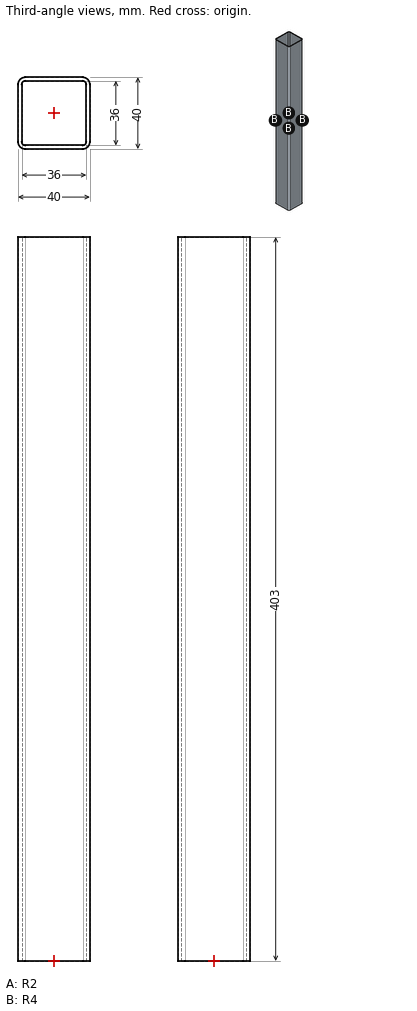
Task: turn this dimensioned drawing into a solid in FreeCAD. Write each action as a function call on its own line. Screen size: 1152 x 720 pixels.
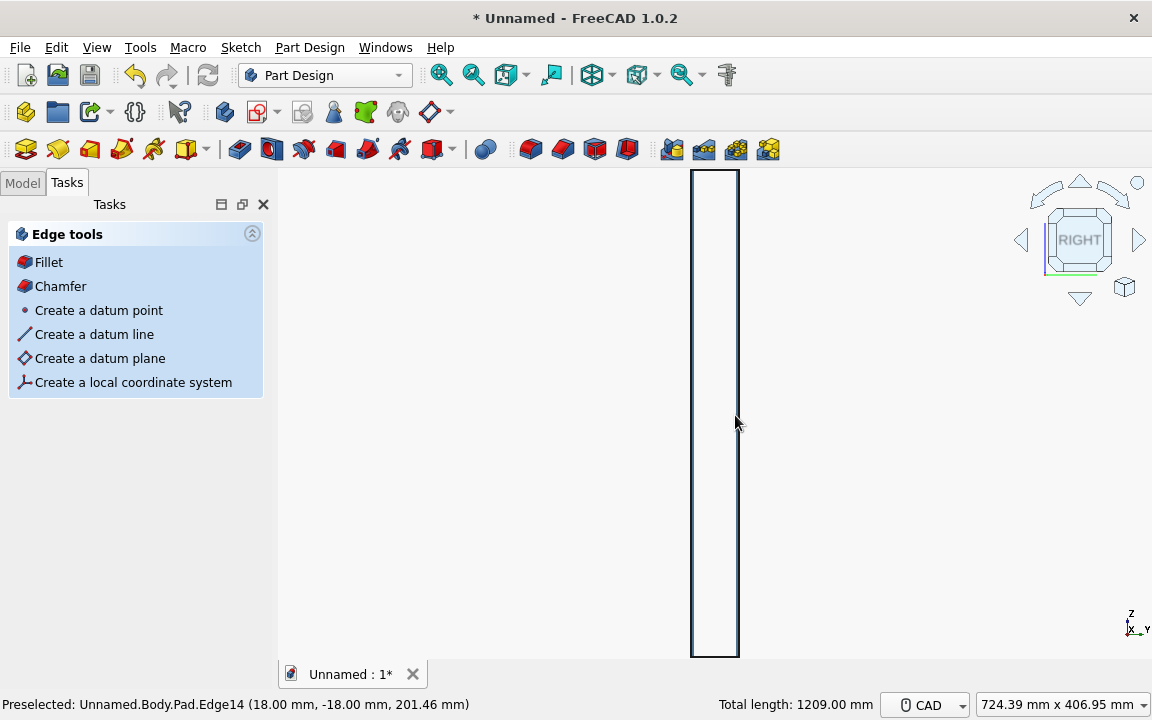
scroll(737, 412, up, 6)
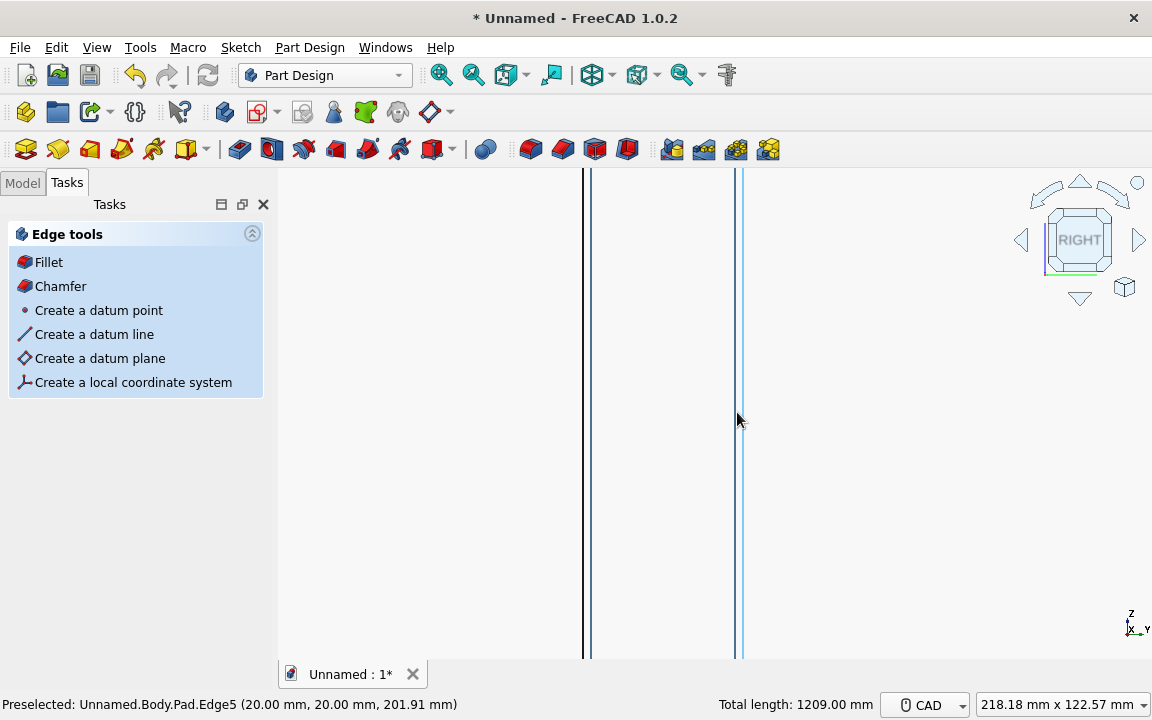
key(v)
key(f)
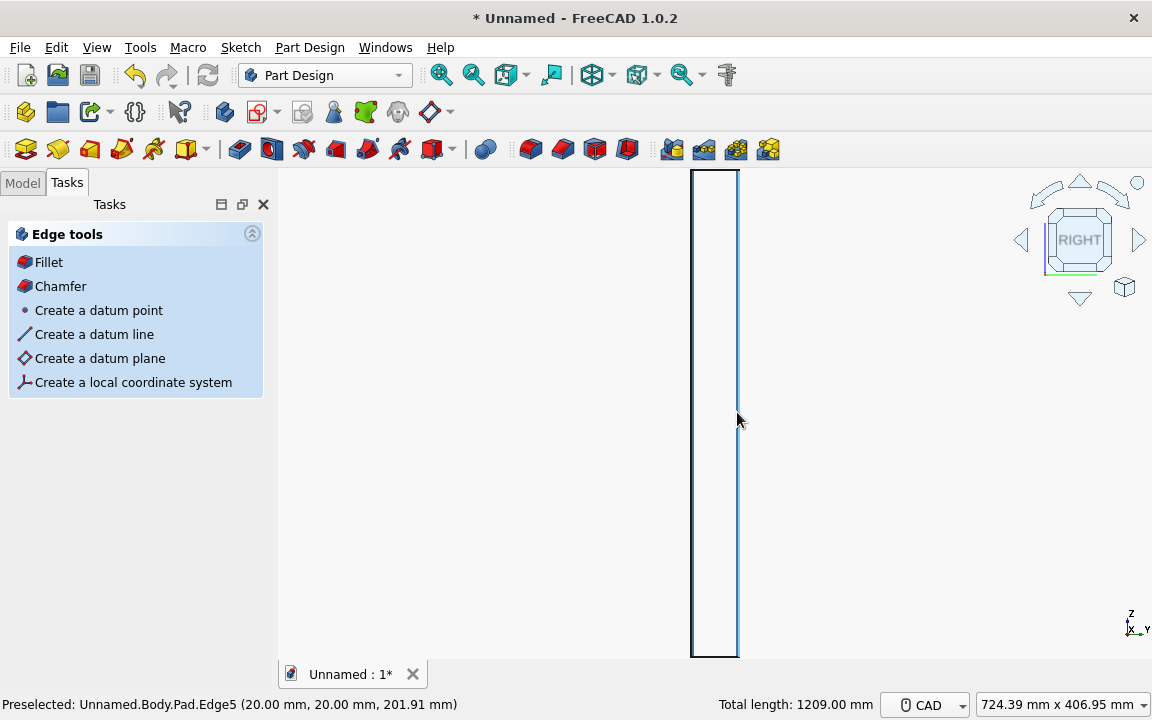
key(5)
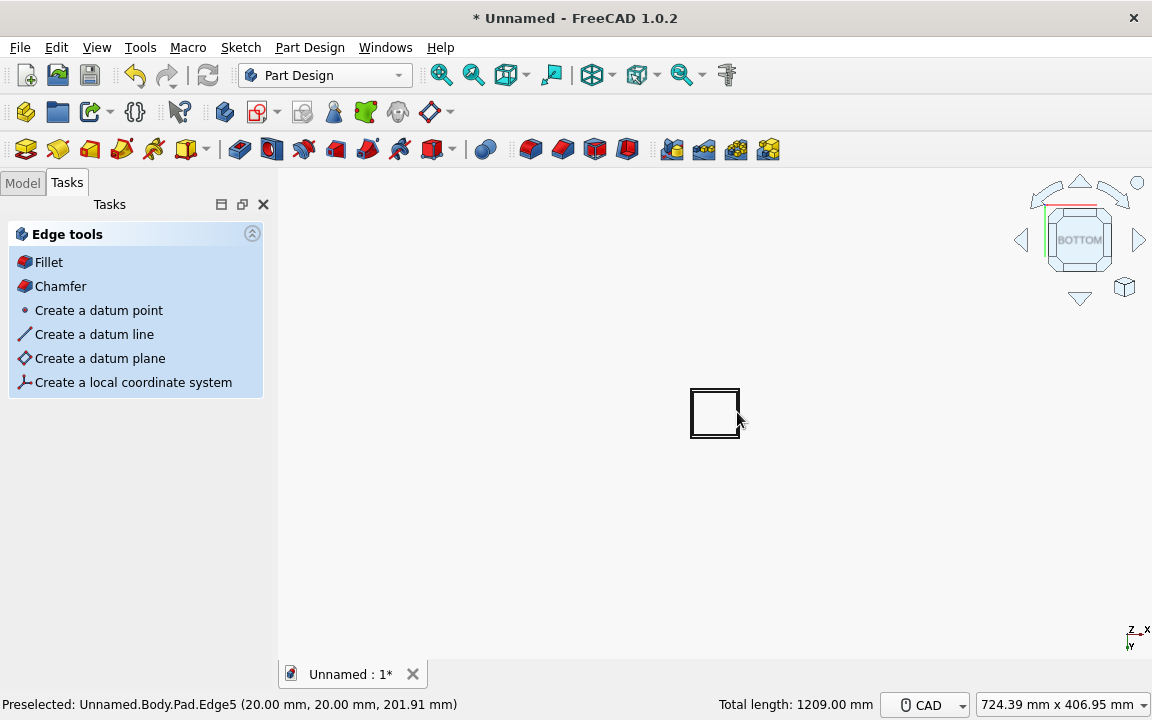
key(v)
key(f)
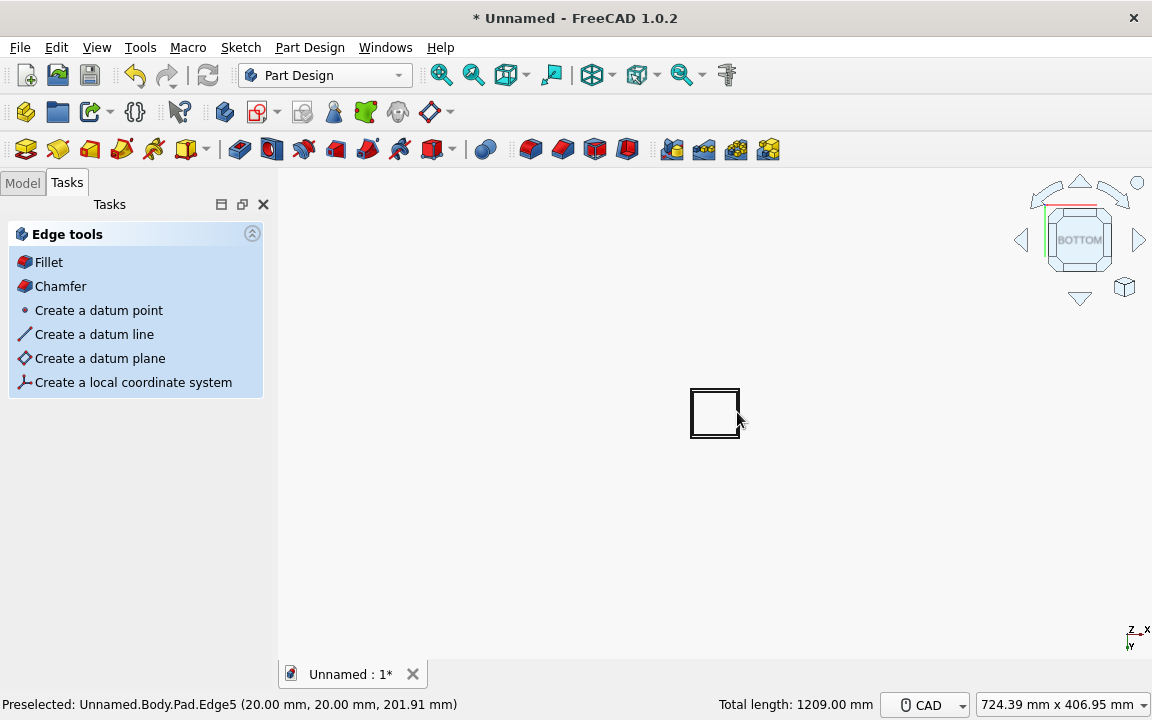
scroll(693, 434, up, 6)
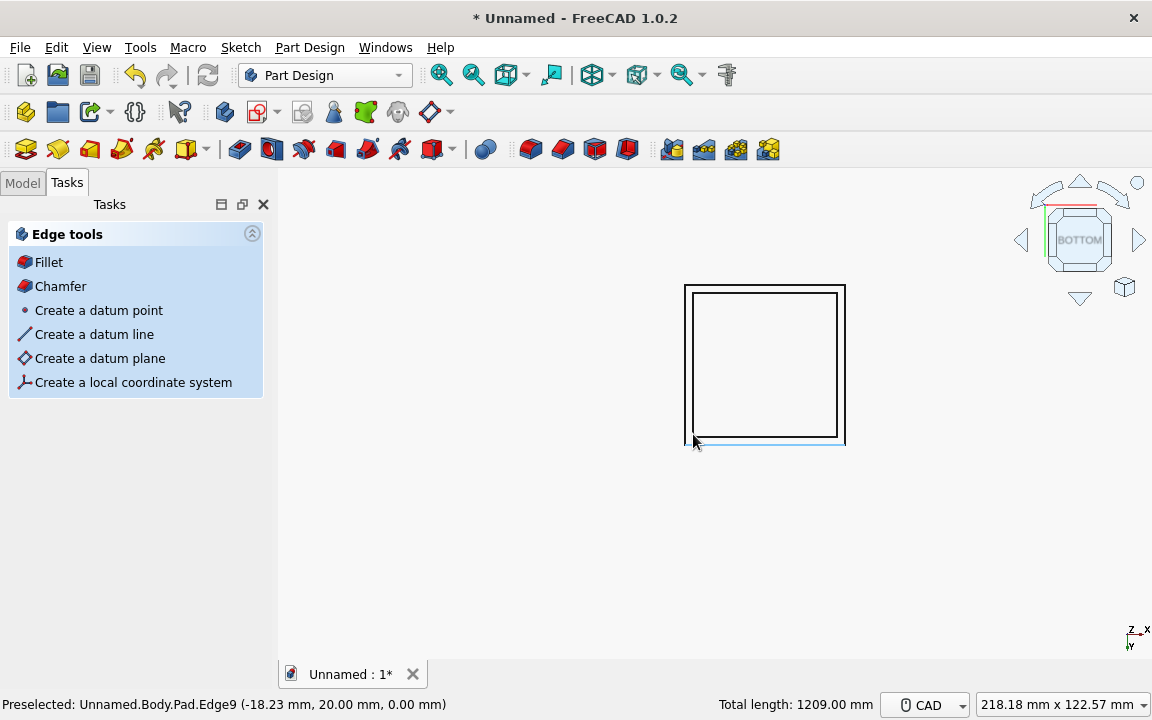
click(442, 76)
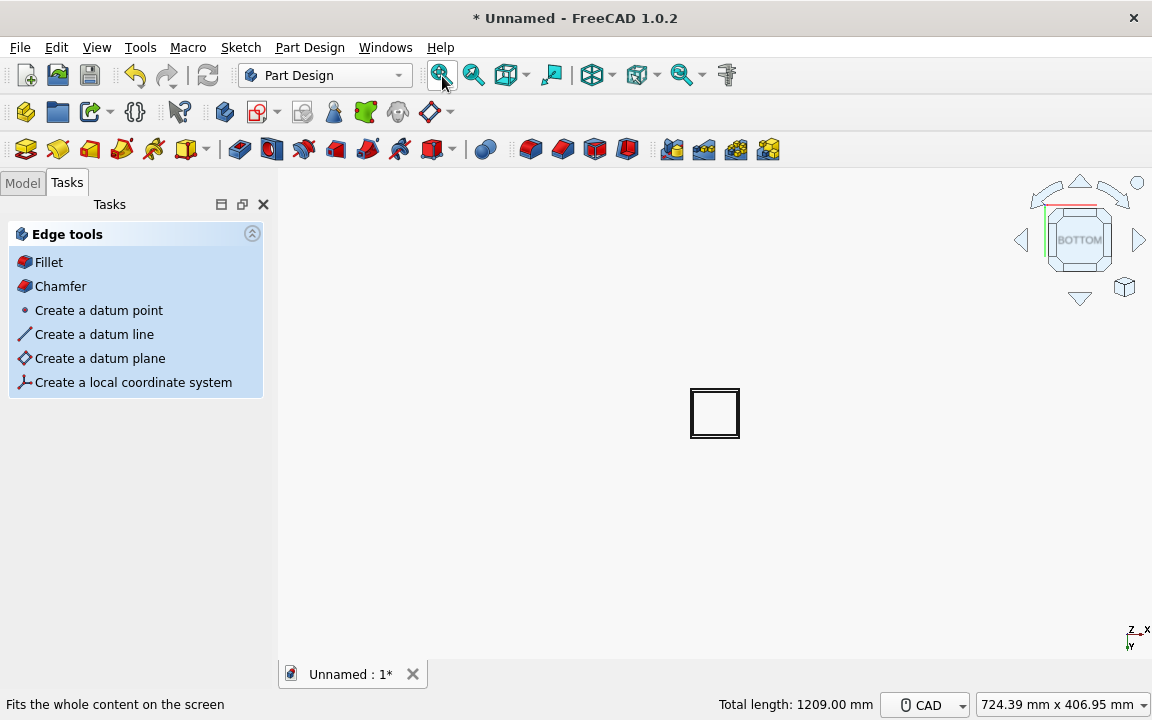
key(4)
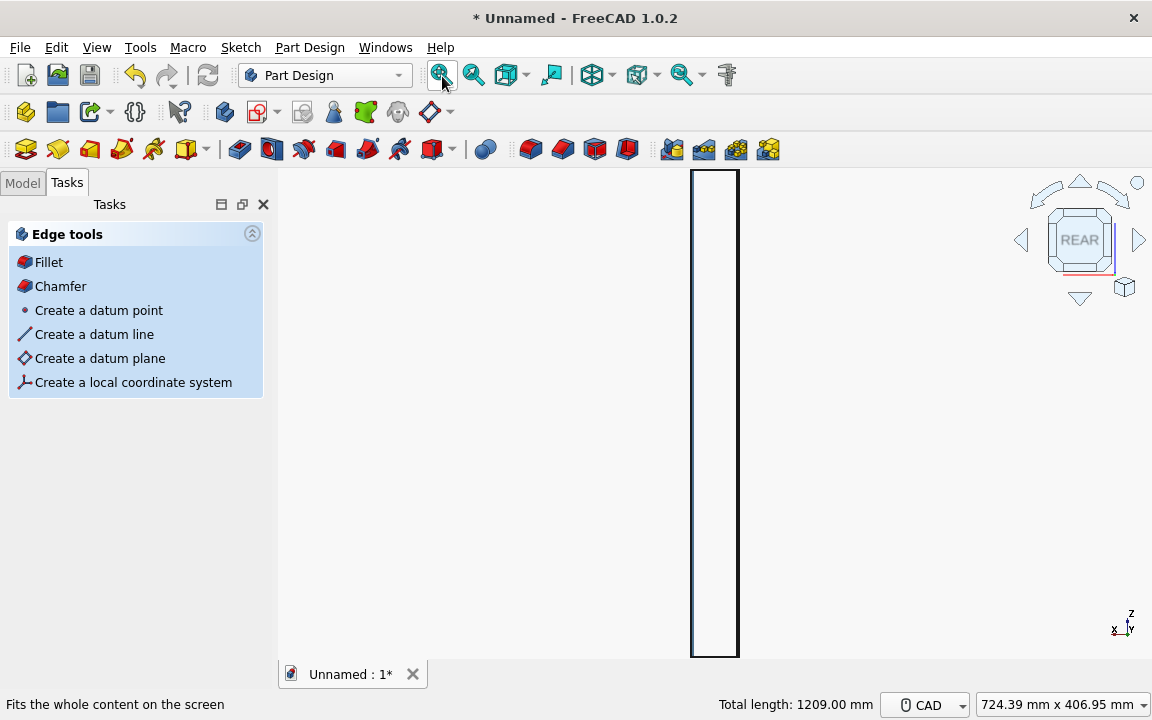
scroll(737, 412, up, 6)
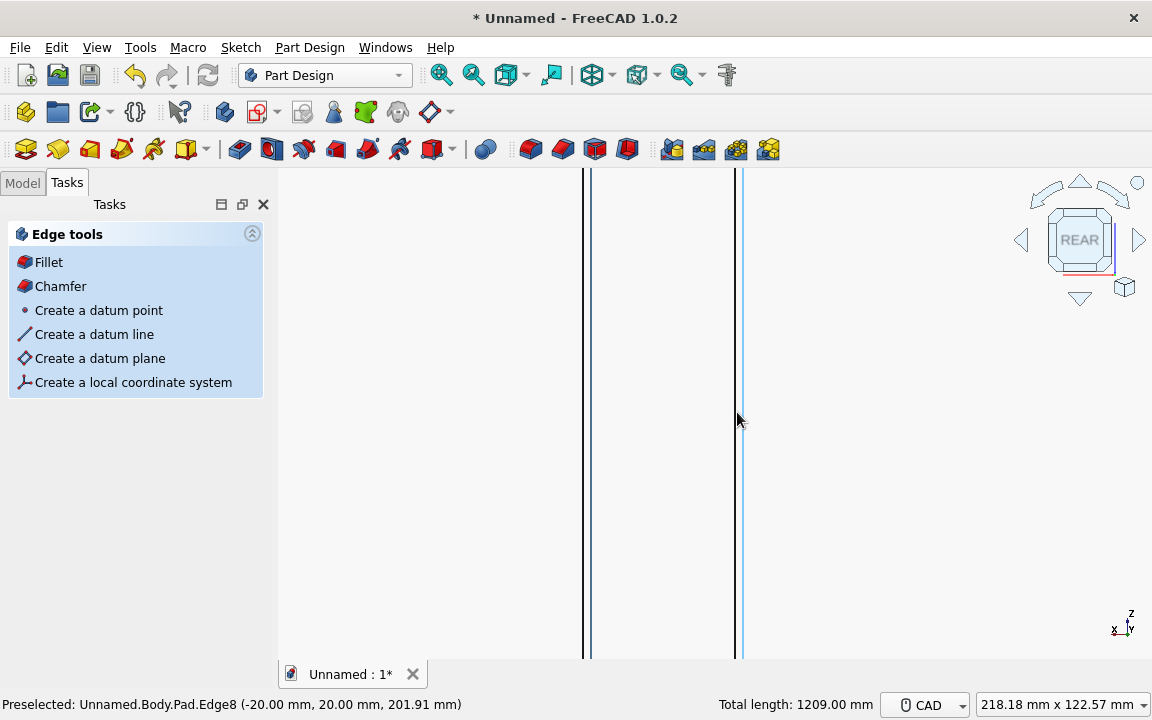
click(735, 415, ctrl)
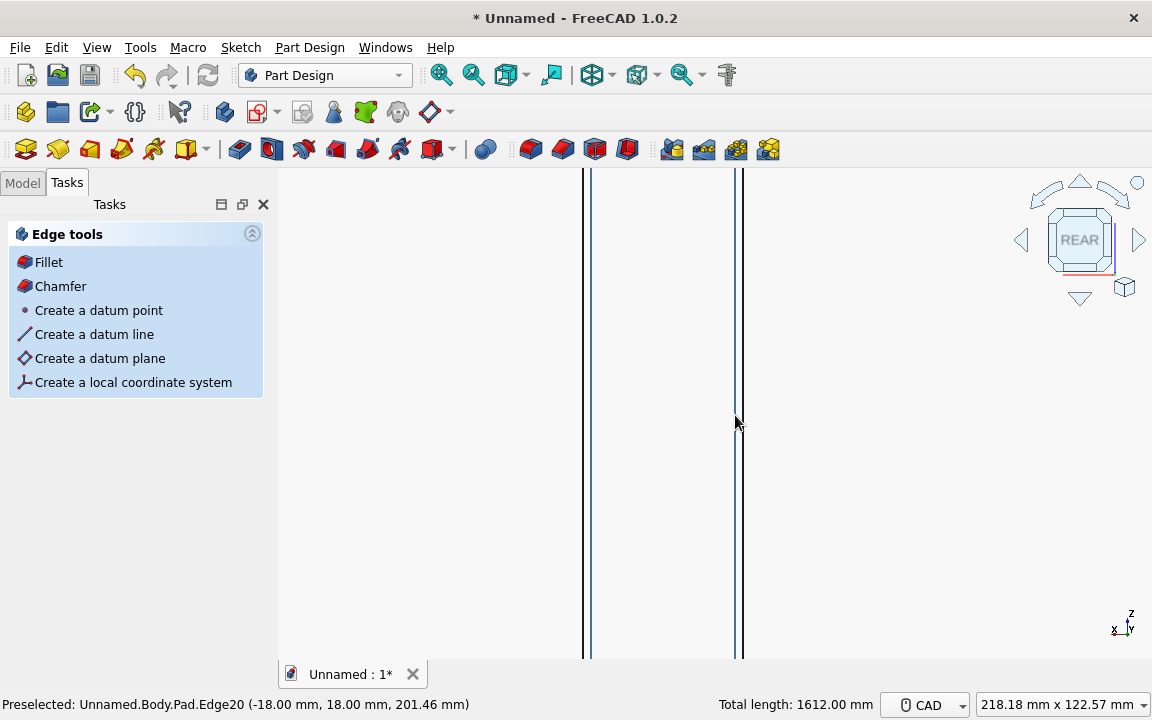
key(v)
key(1)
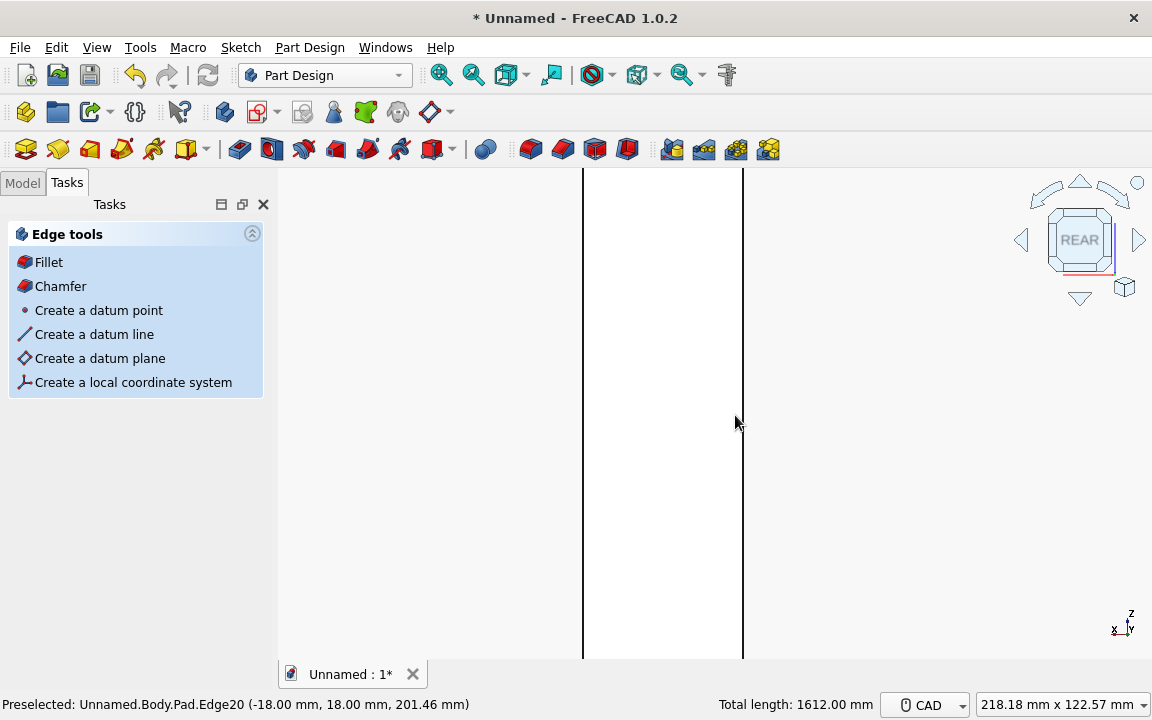
click(532, 150)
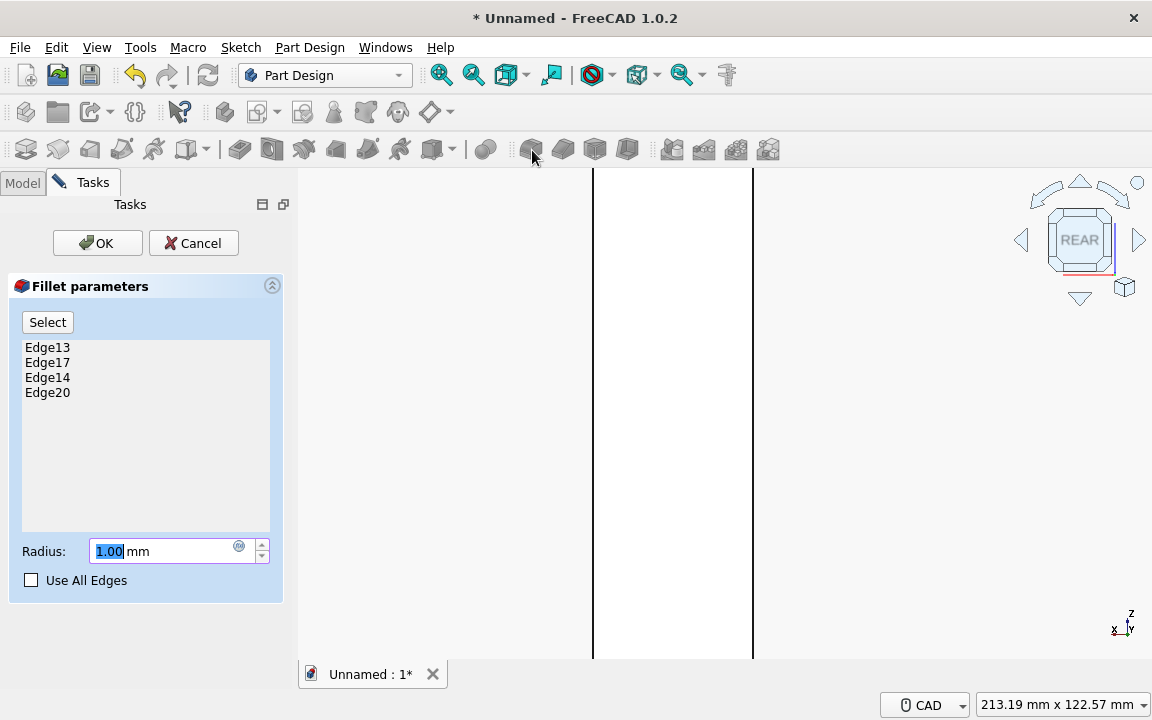
text(2)
key(Tab)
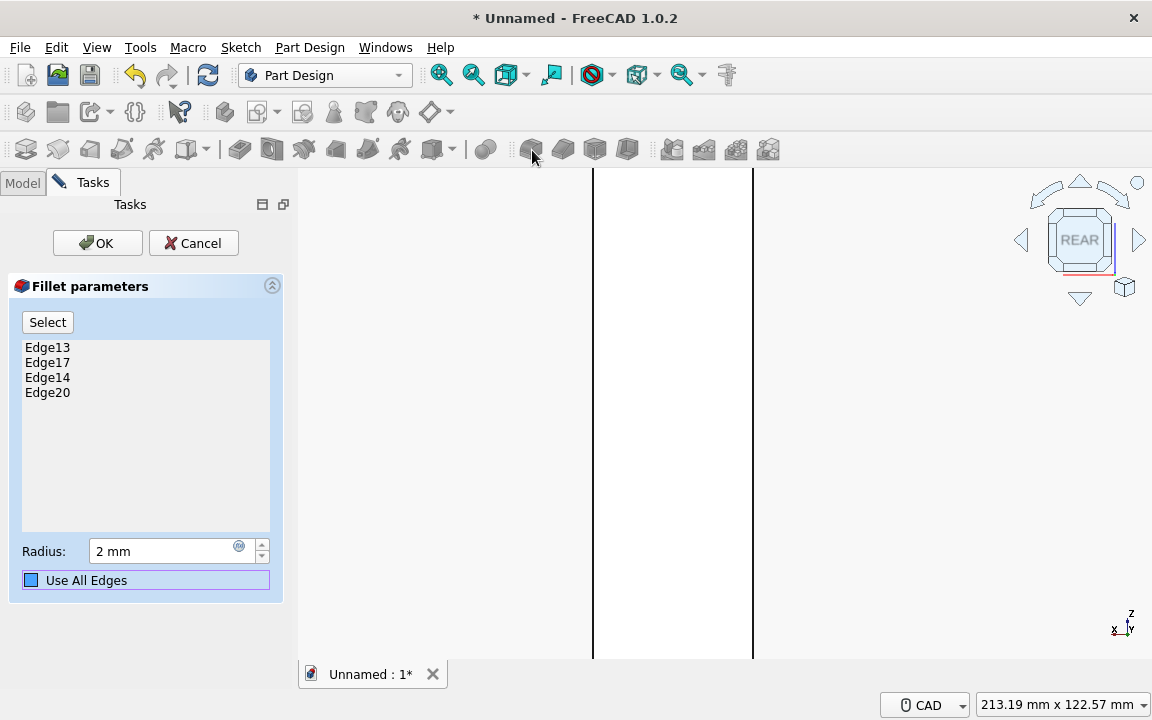
click(98, 243)